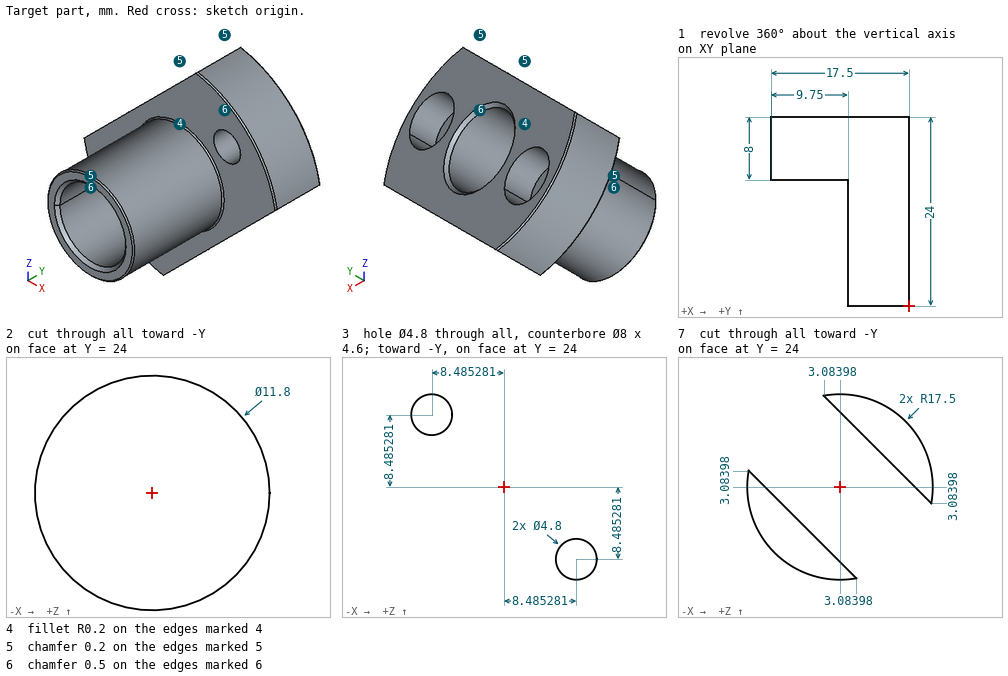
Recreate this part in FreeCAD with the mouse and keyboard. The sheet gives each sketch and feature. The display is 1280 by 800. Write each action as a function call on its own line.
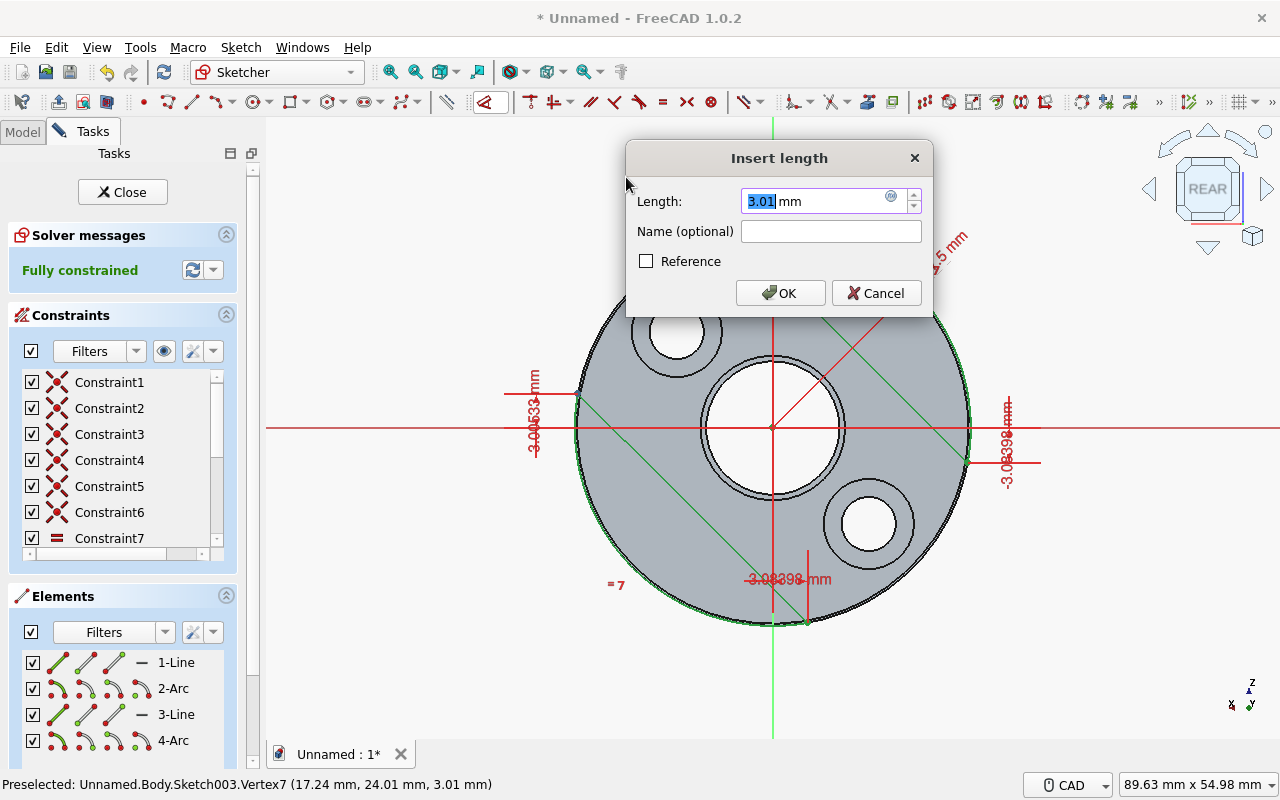
text(3.08398)
key(Return)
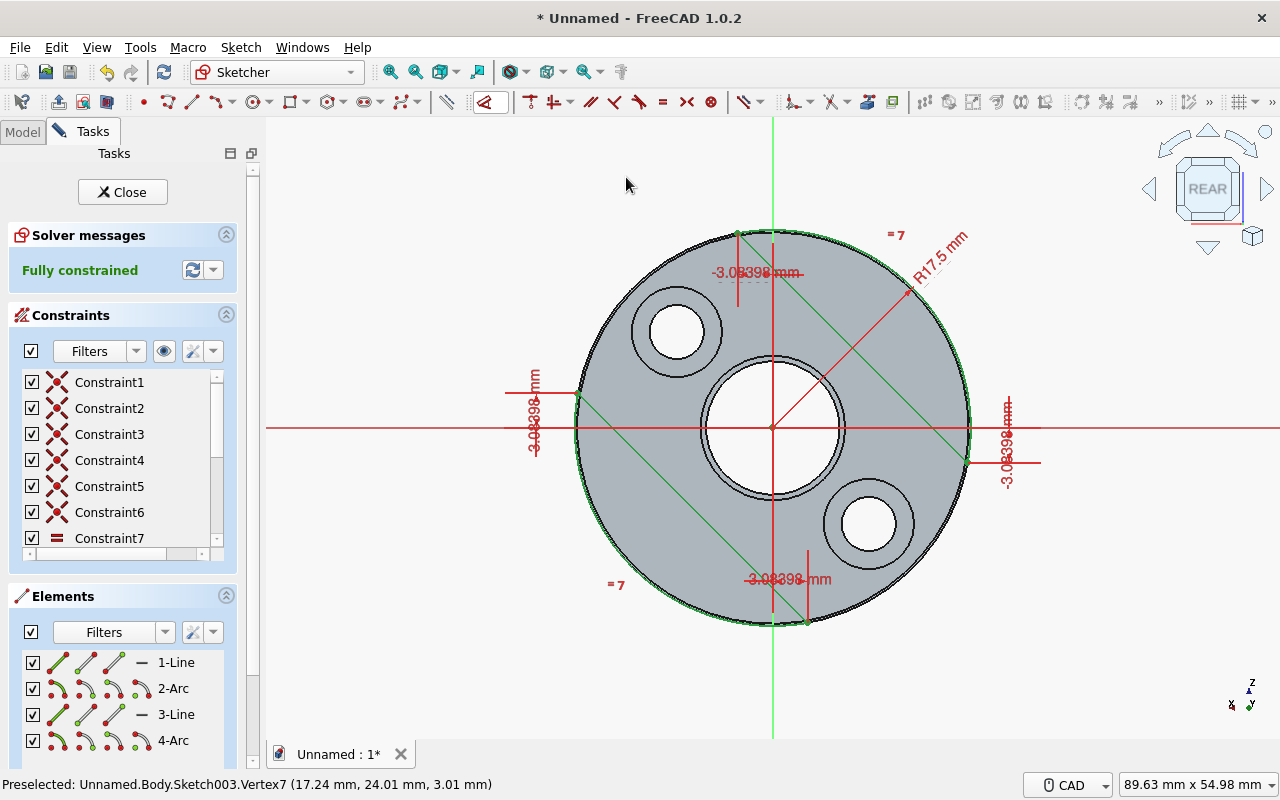
click(123, 192)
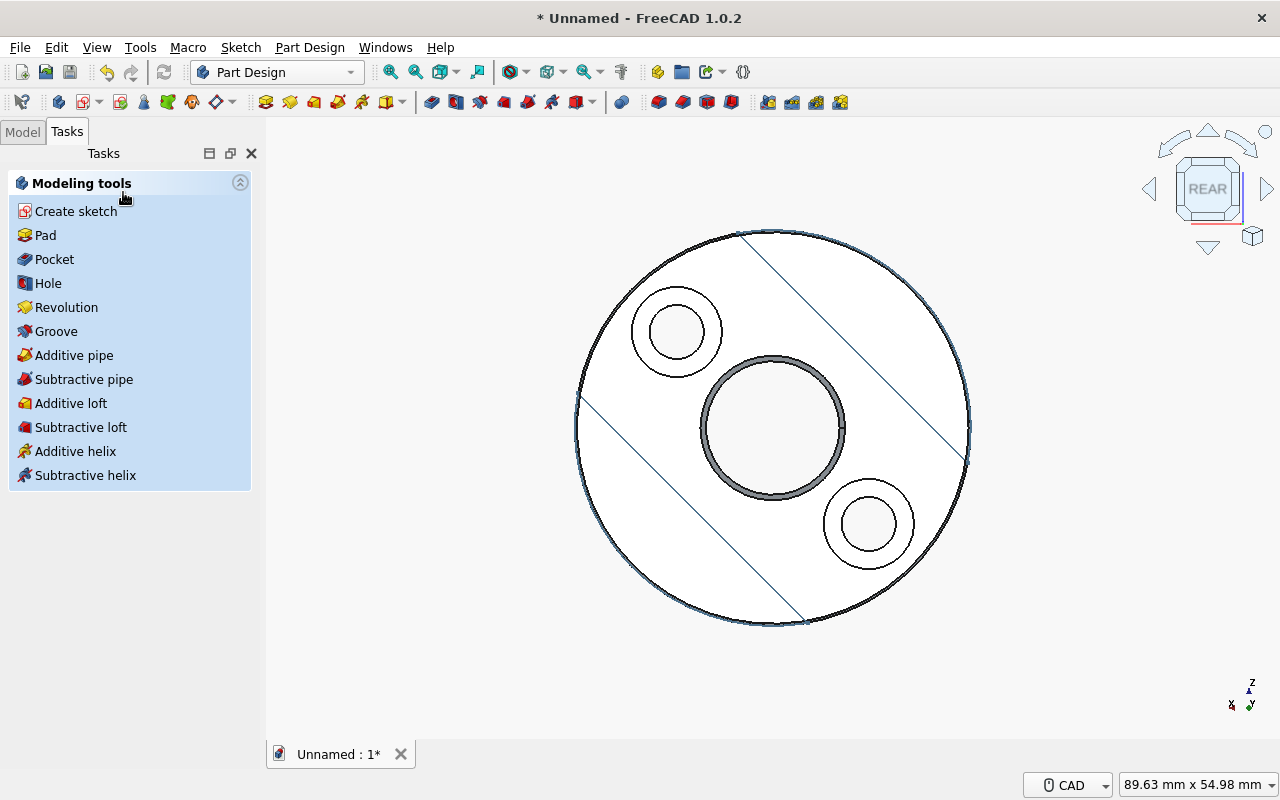
click(432, 102)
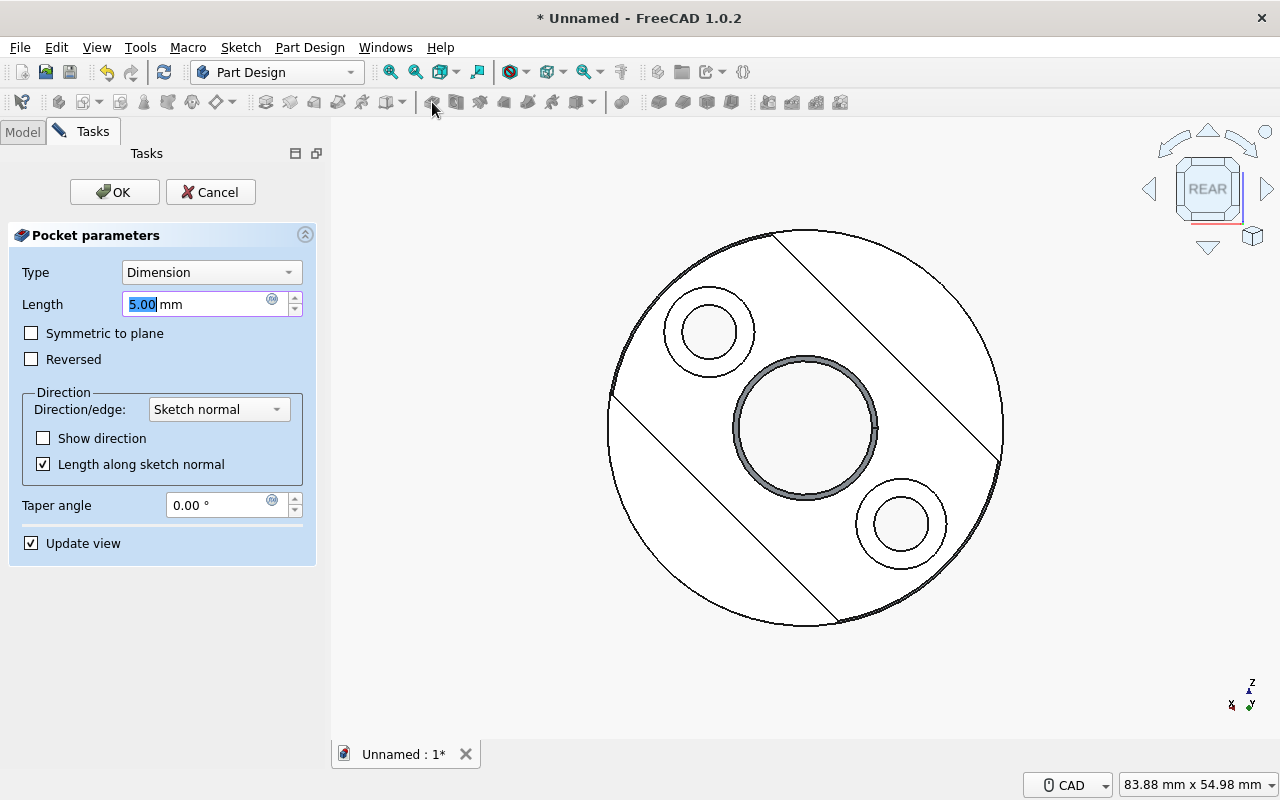
click(212, 272)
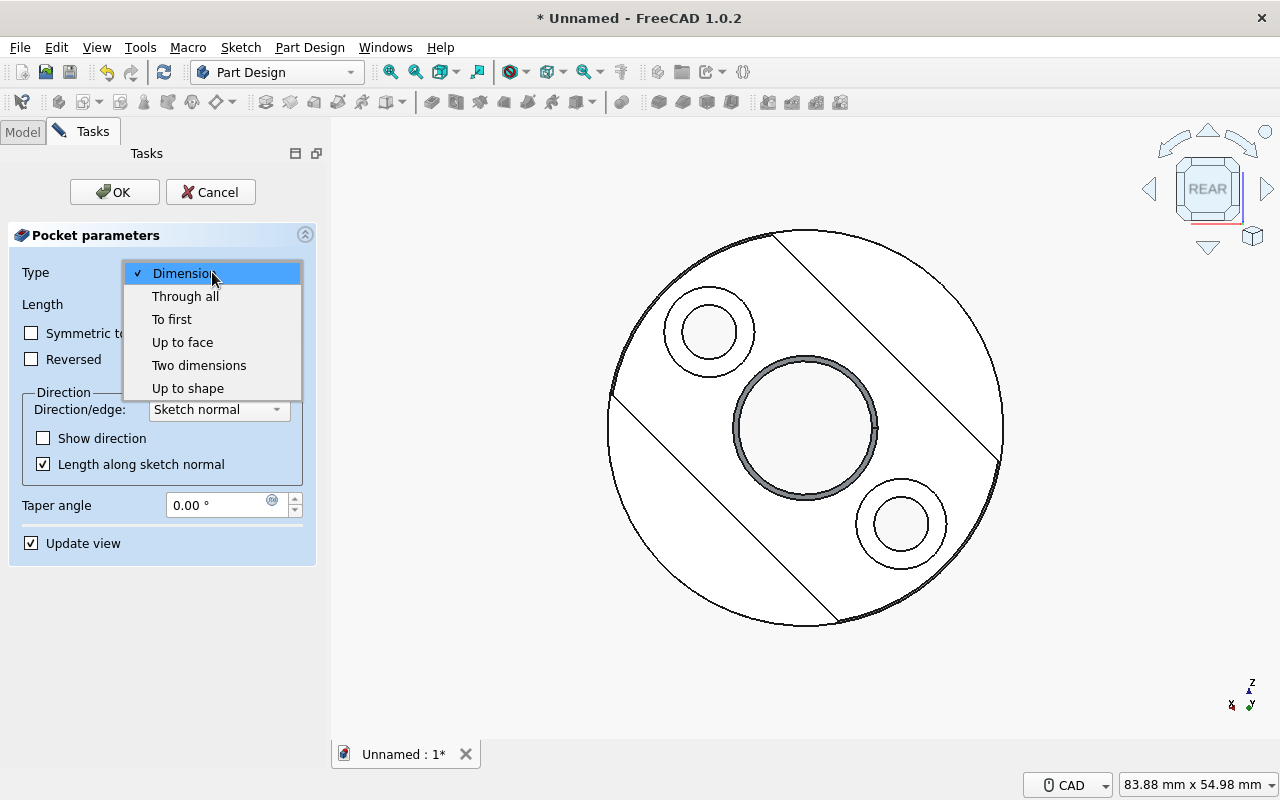
click(212, 296)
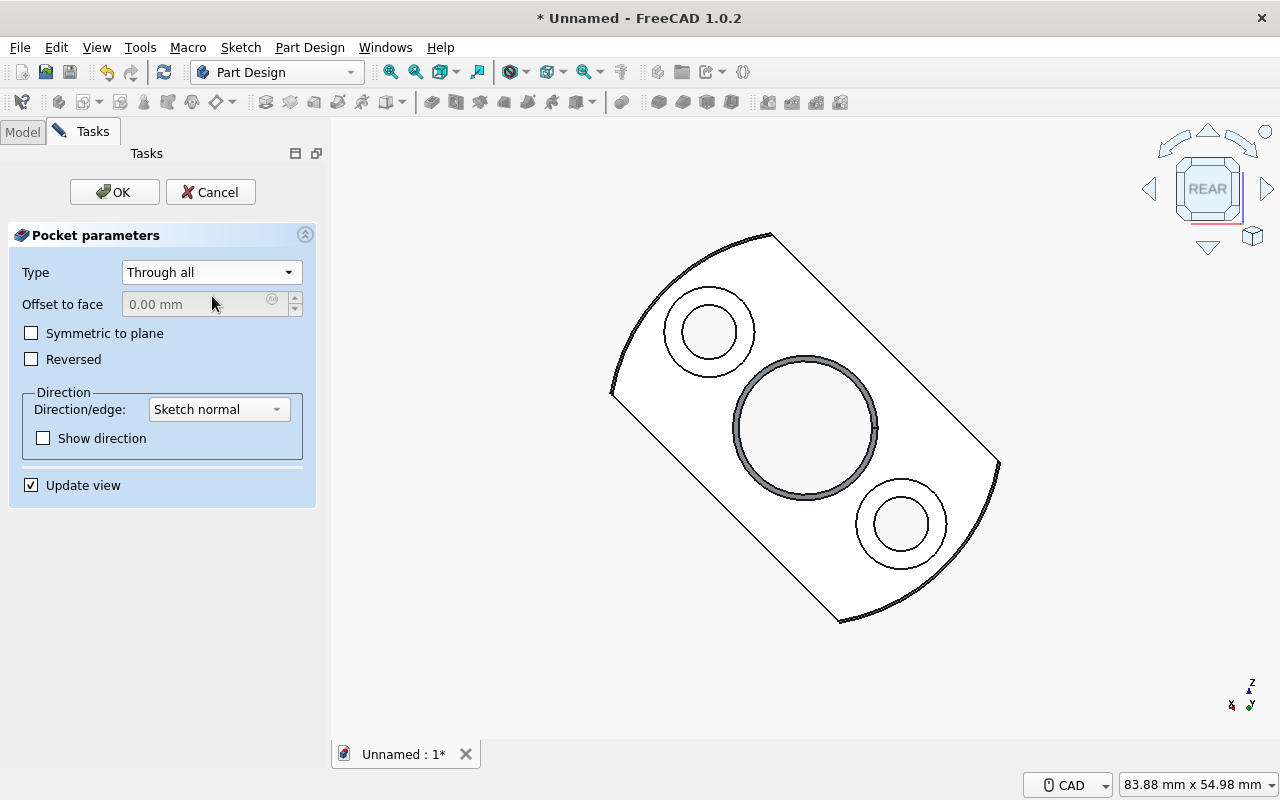
click(115, 192)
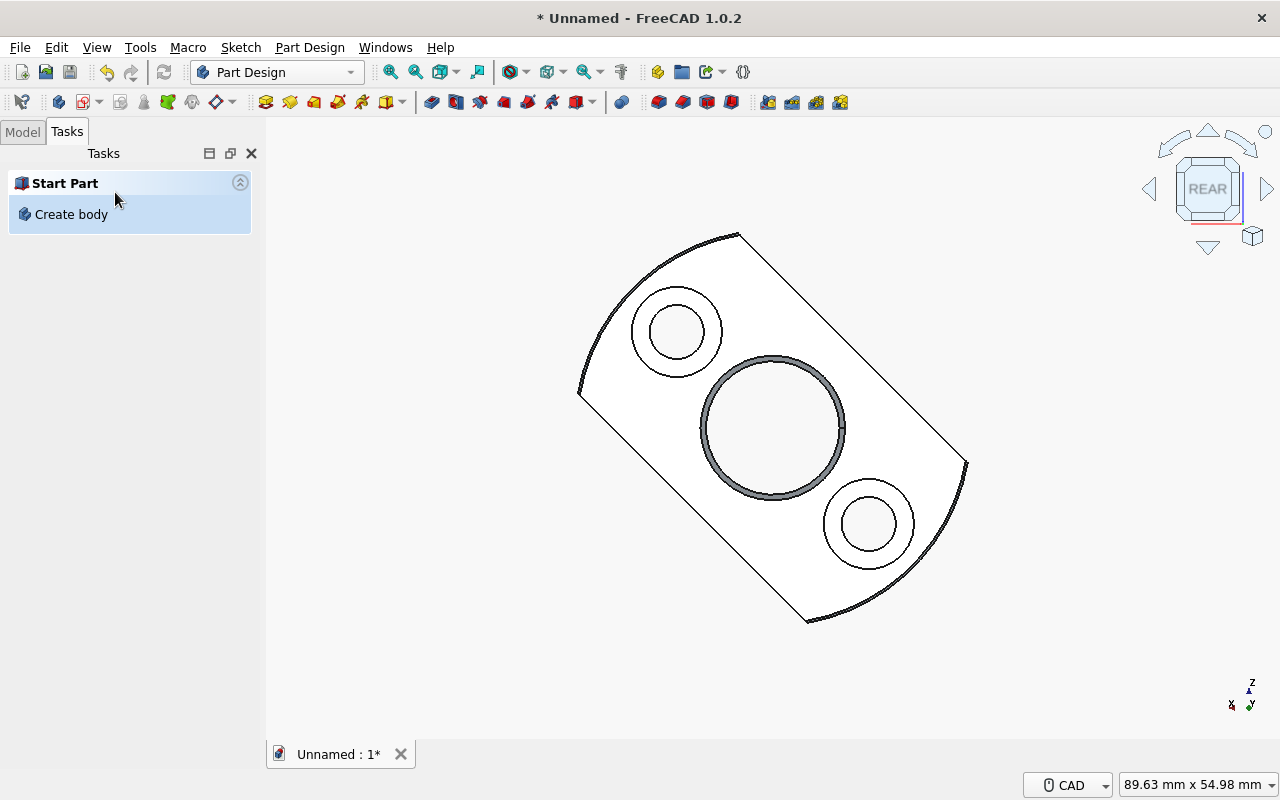
key(0)